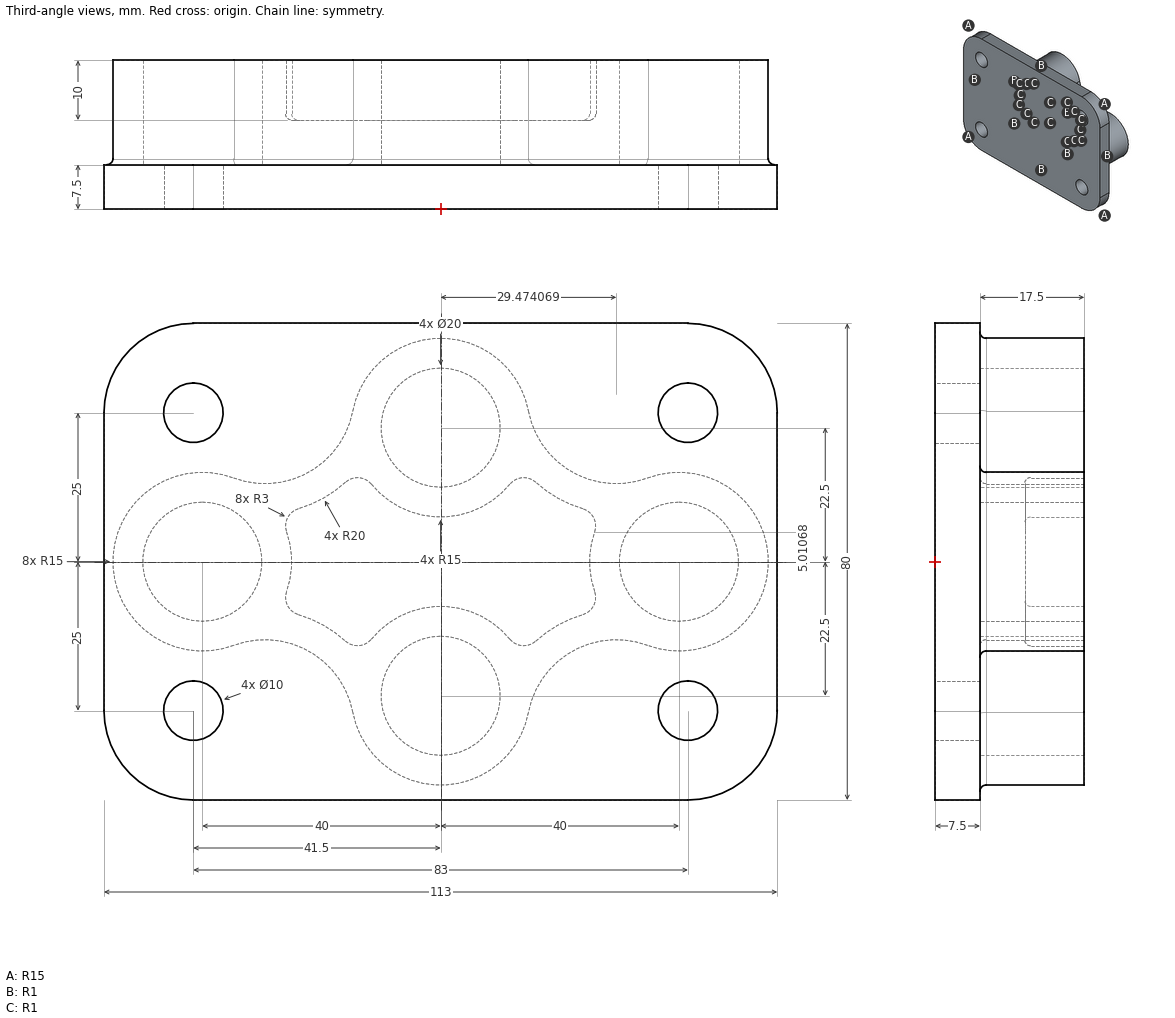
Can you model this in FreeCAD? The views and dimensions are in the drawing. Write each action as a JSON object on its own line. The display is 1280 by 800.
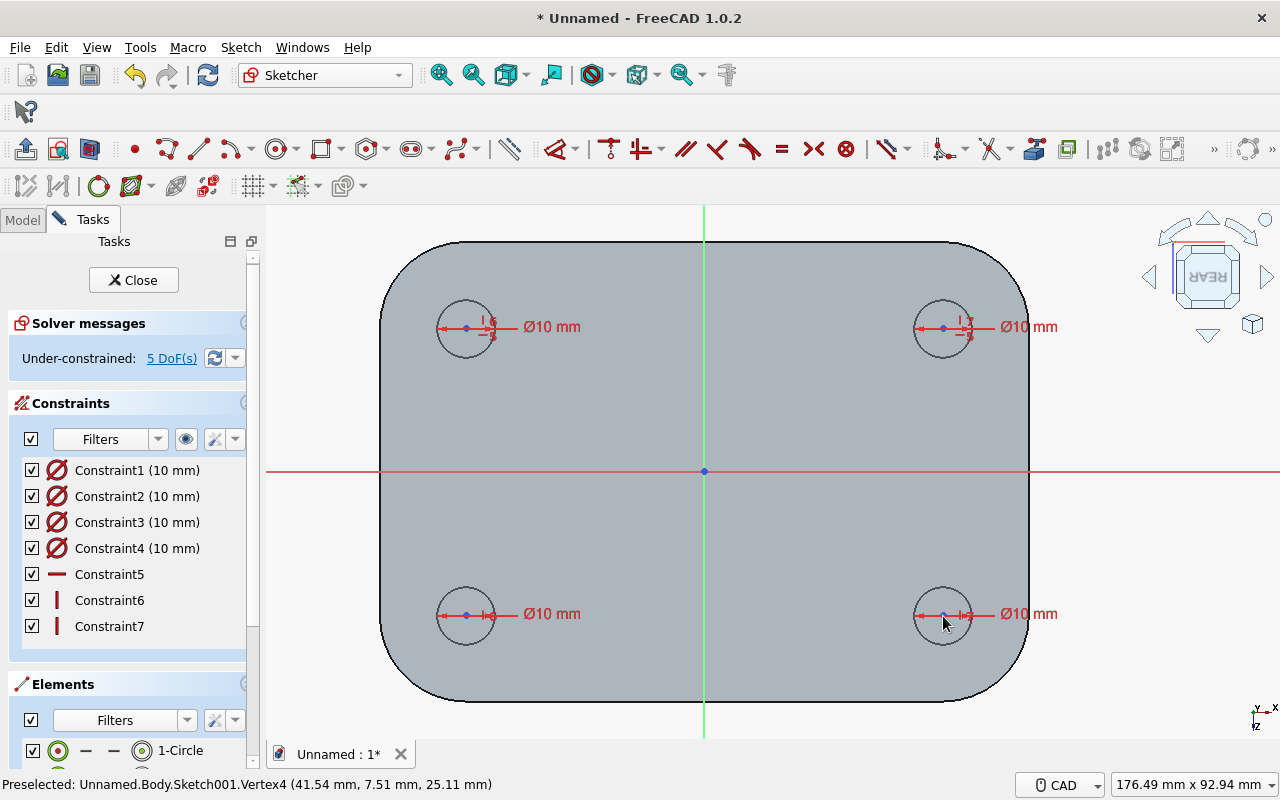
{"action": "left_click", "coordinate": [466, 616]}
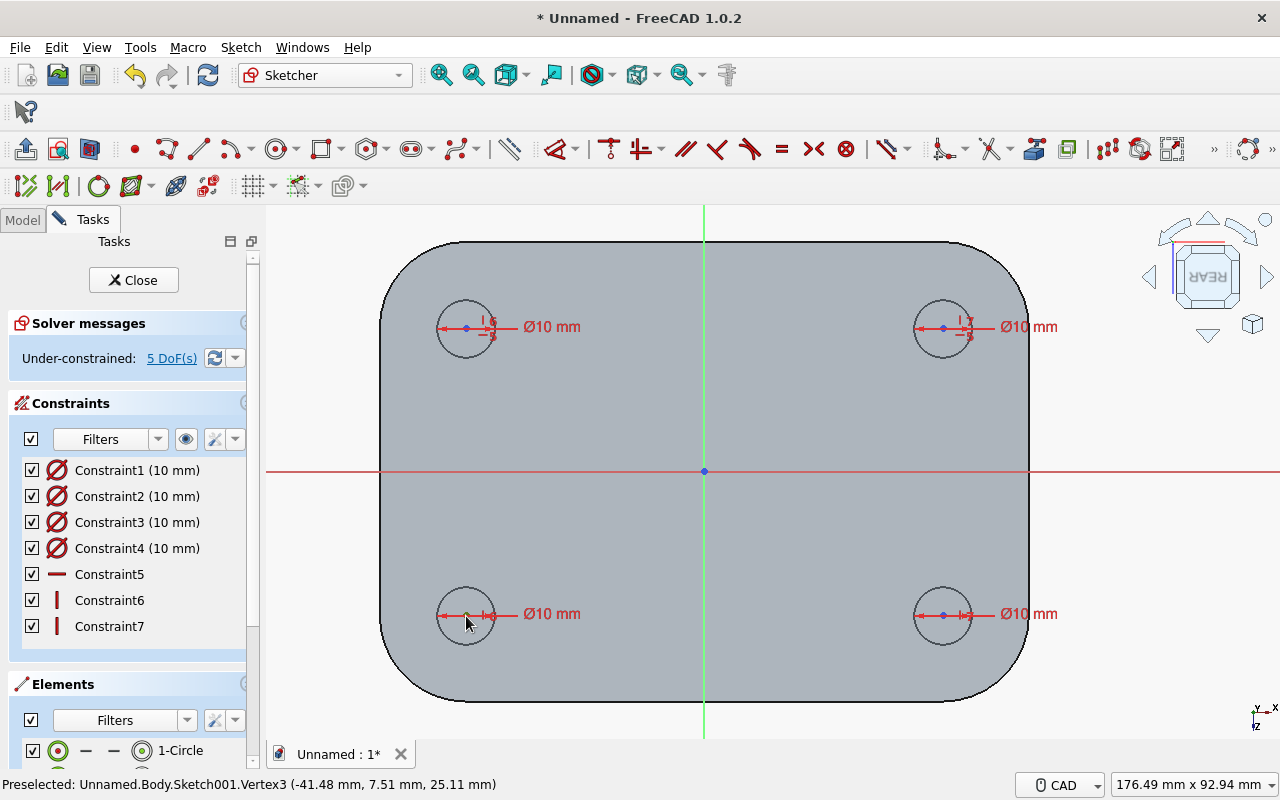
{"action": "left_click", "coordinate": [943, 616]}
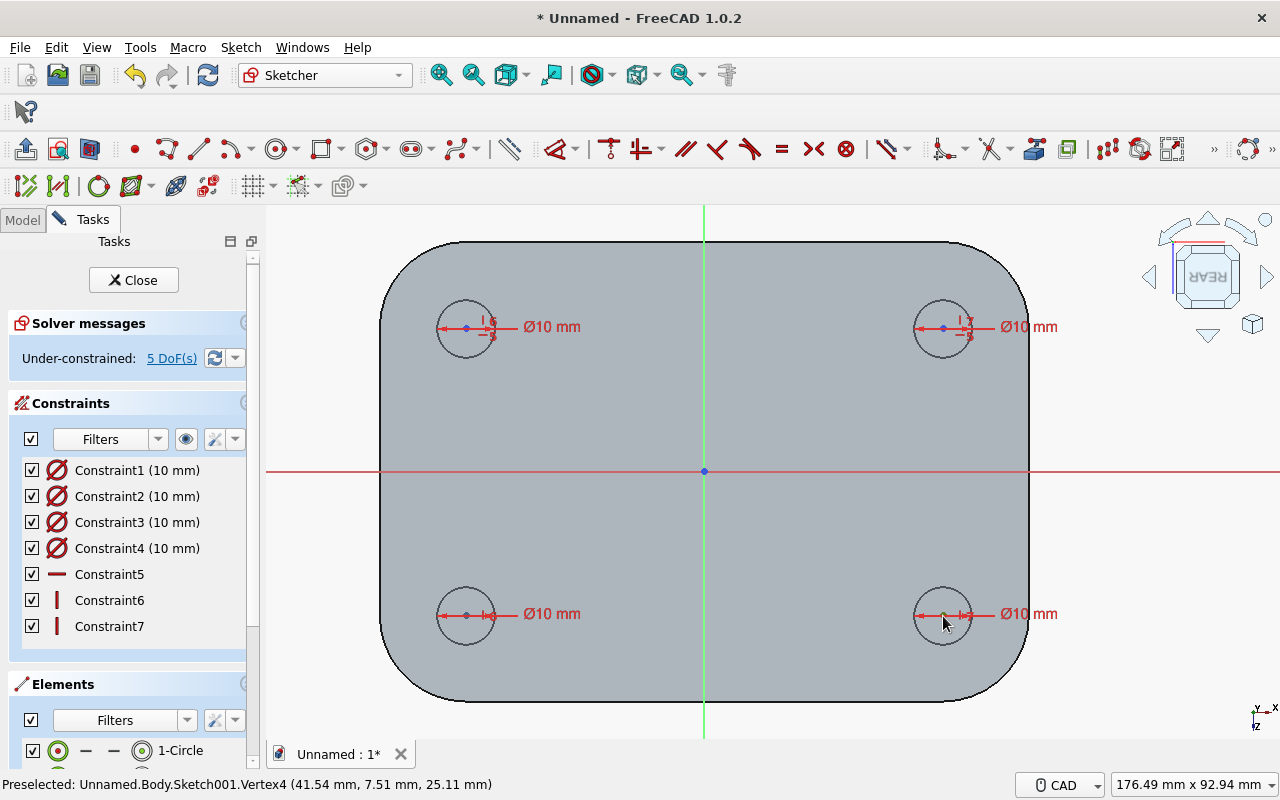
{"action": "left_click", "coordinate": [664, 150]}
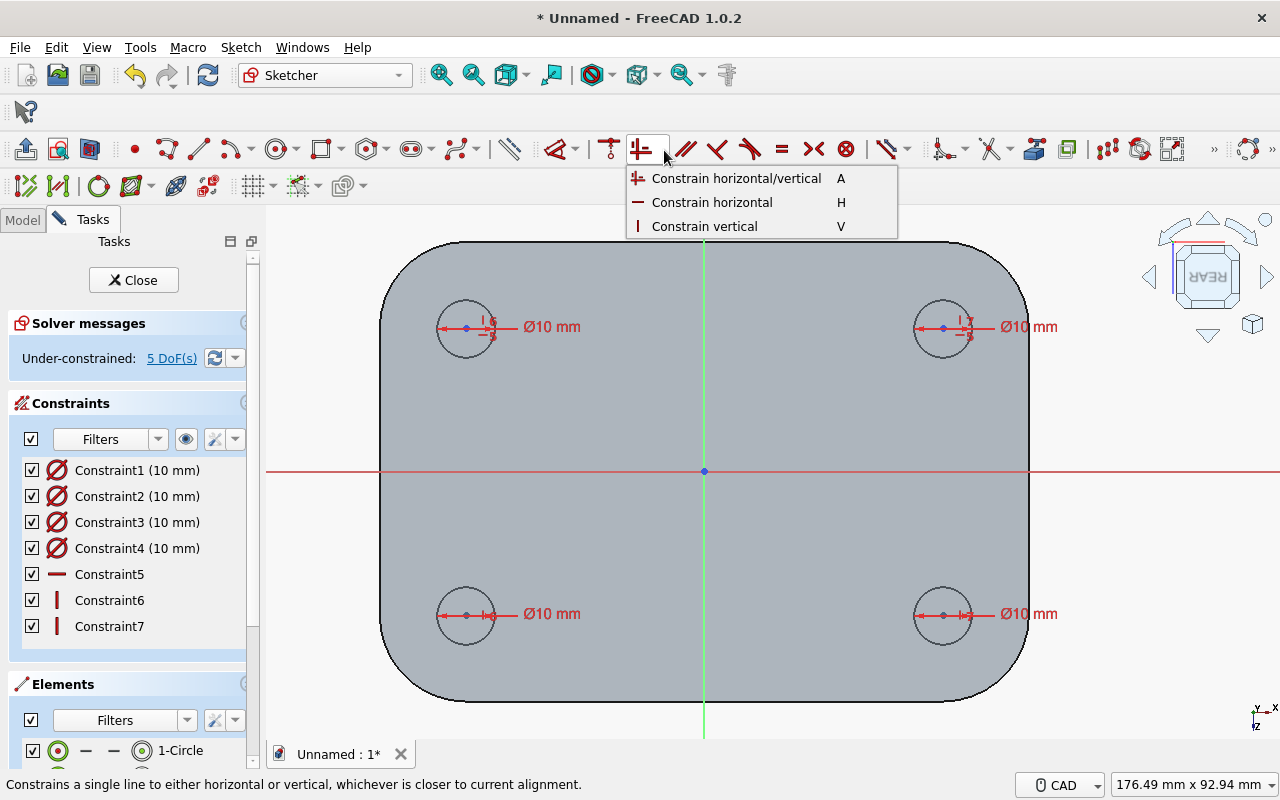
{"action": "left_click", "coordinate": [762, 202]}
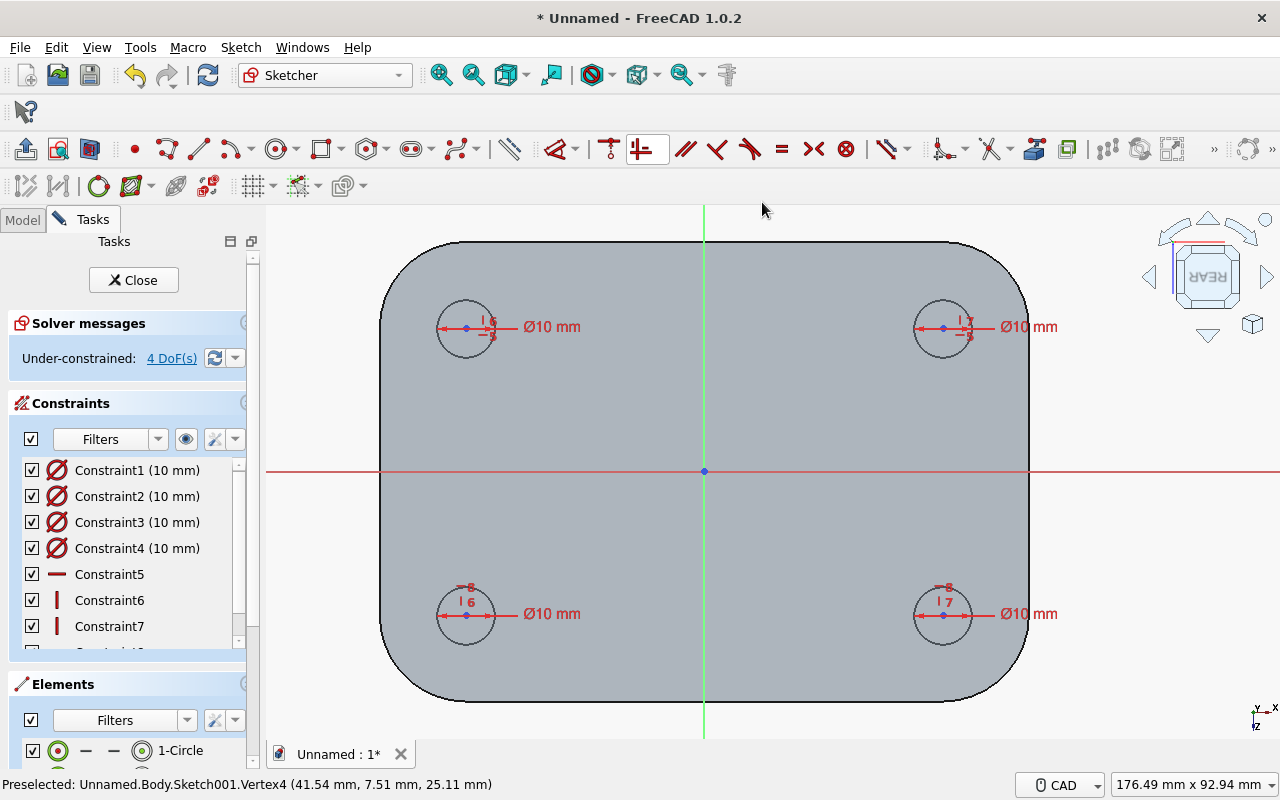
{"action": "key", "text": "d"}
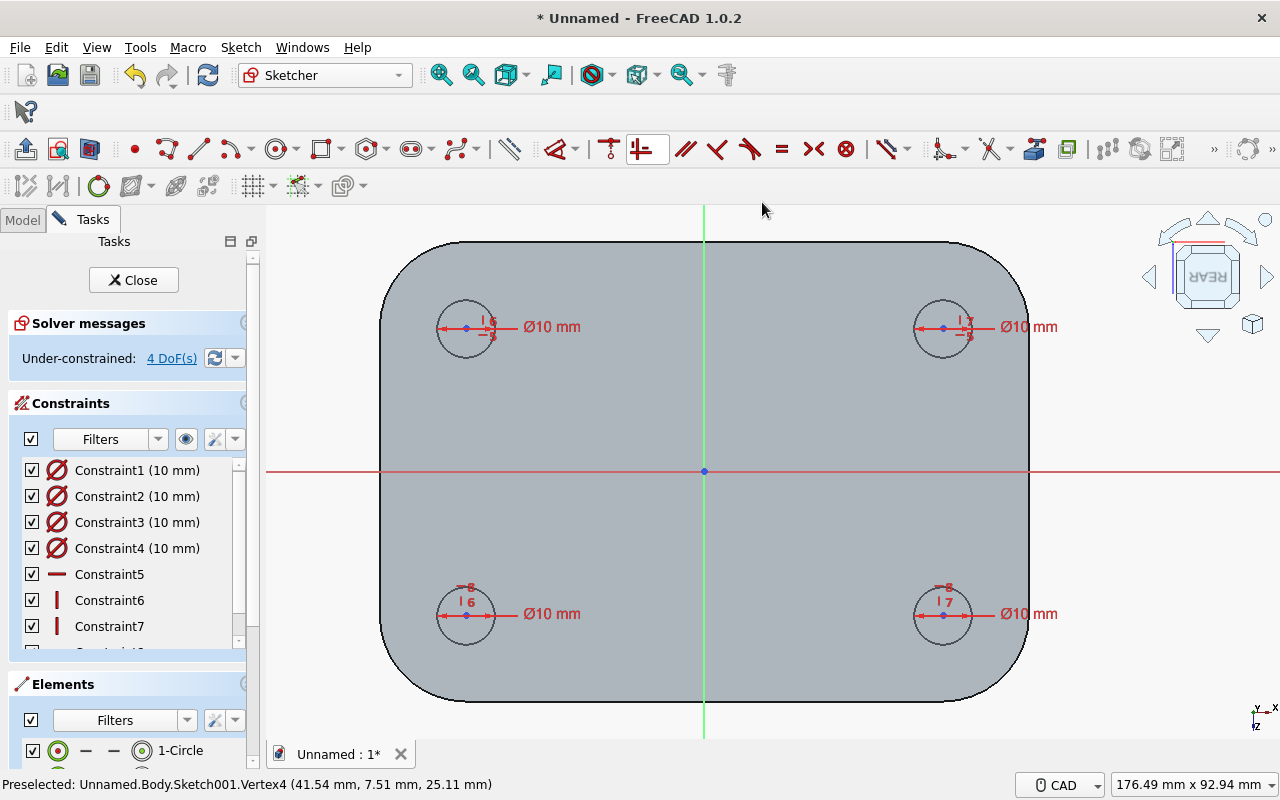
{"action": "left_click", "coordinate": [466, 329]}
{"action": "left_click", "coordinate": [432, 400]}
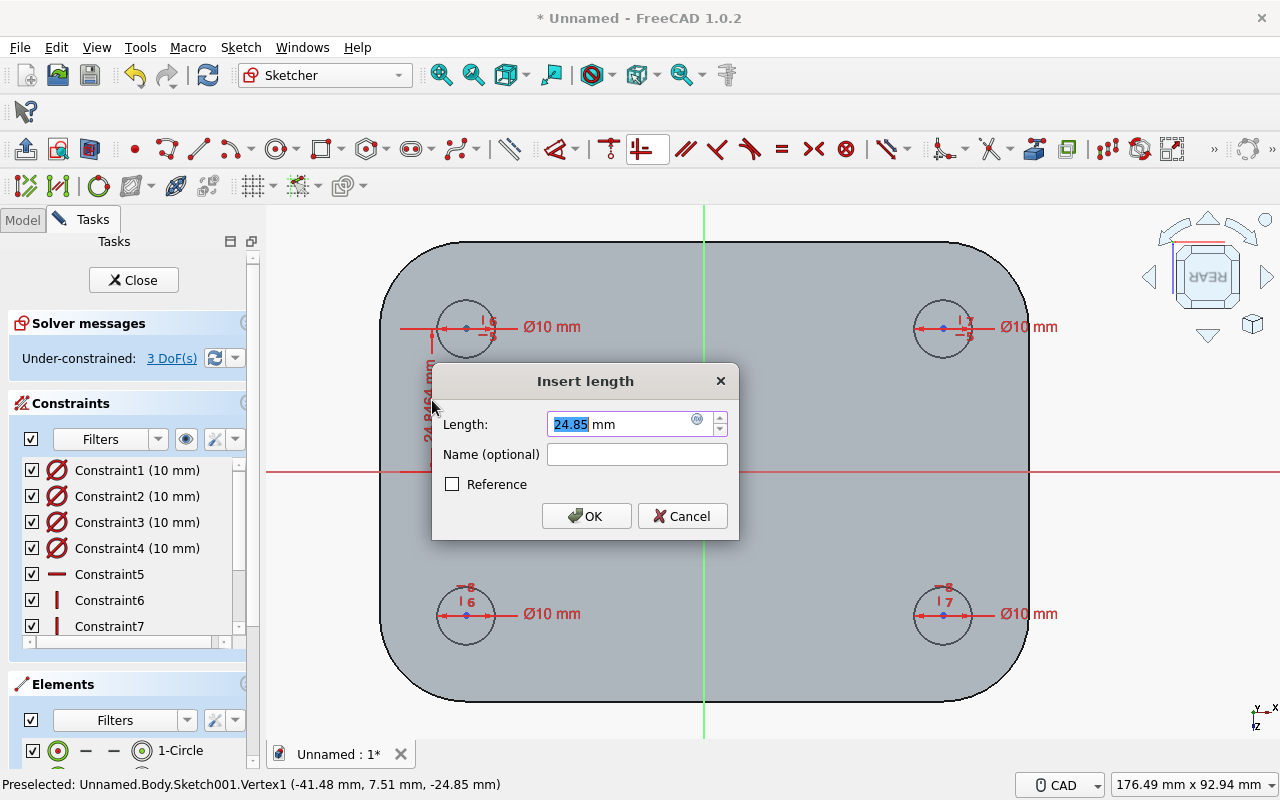
{"action": "type", "text": "25"}
{"action": "key", "text": "Return"}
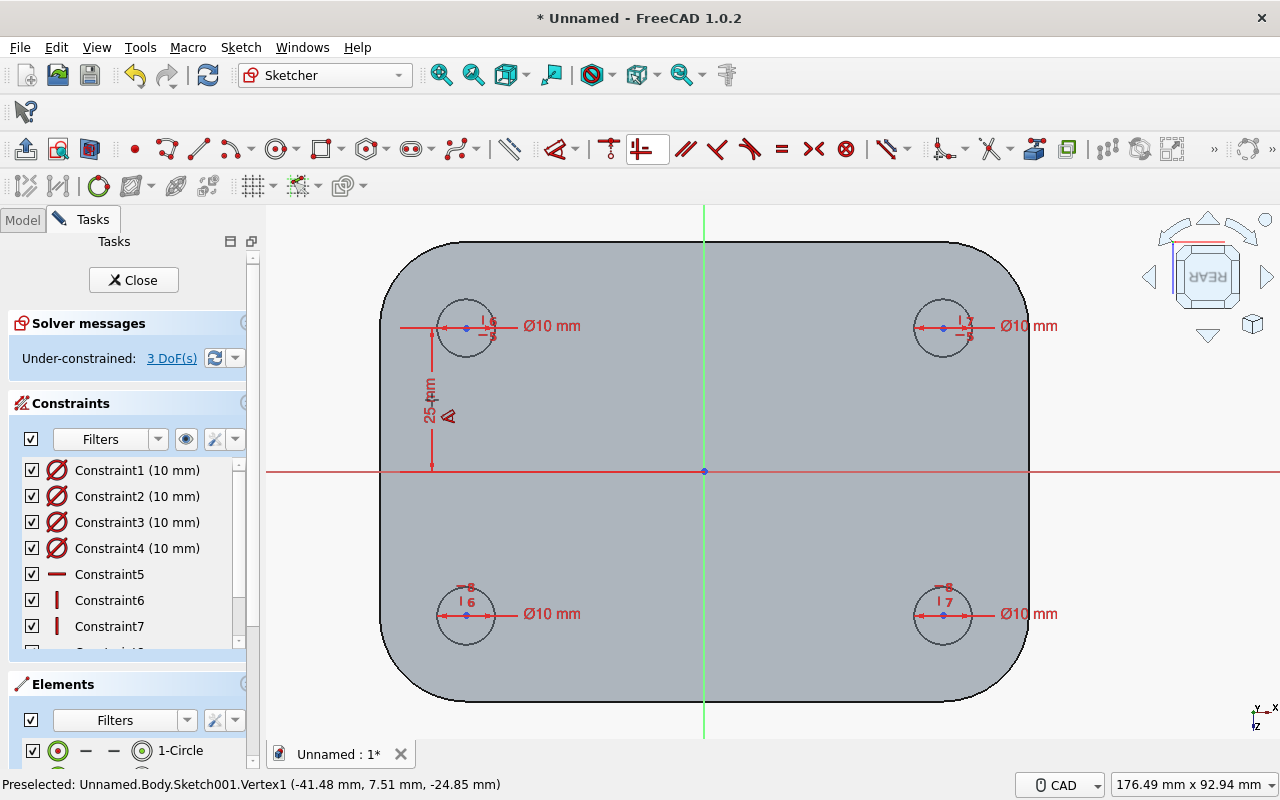
{"action": "left_click", "coordinate": [466, 616]}
{"action": "left_click", "coordinate": [432, 544]}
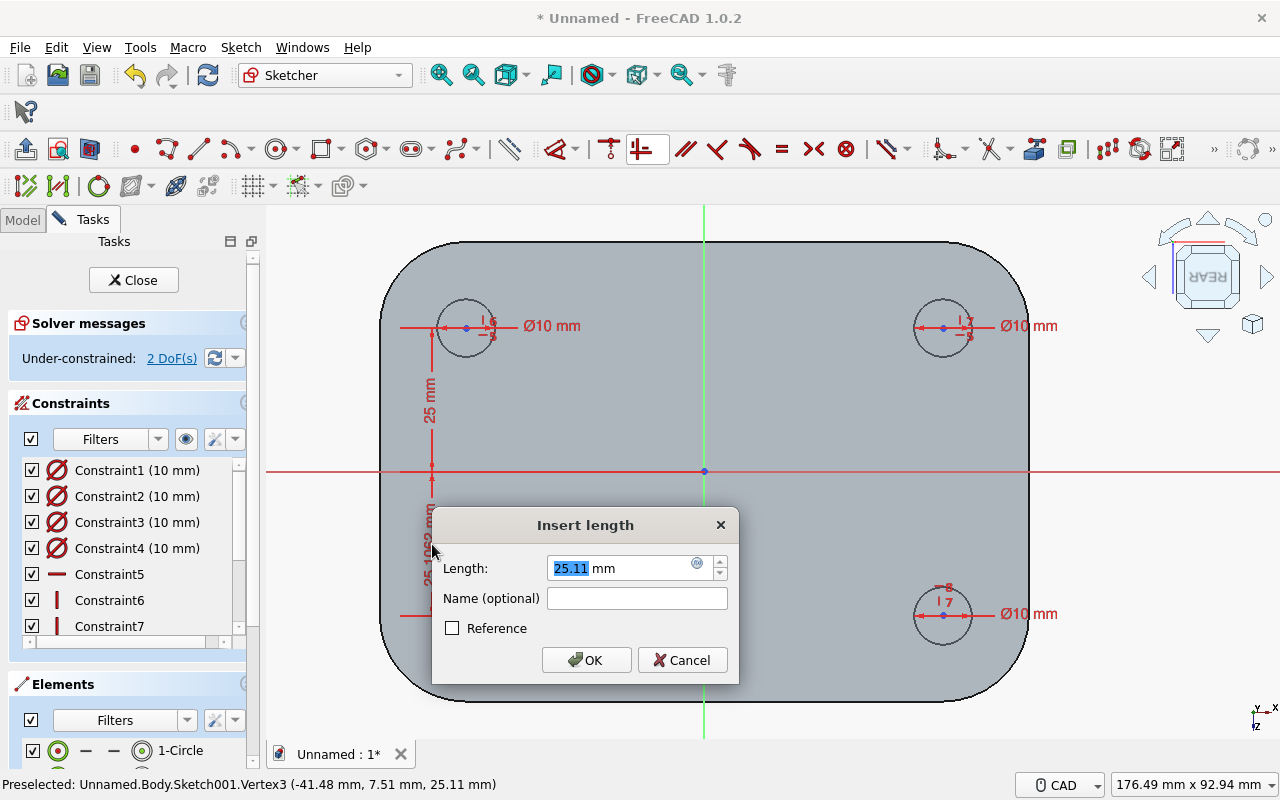
{"action": "type", "text": "25"}
{"action": "key", "text": "Return"}